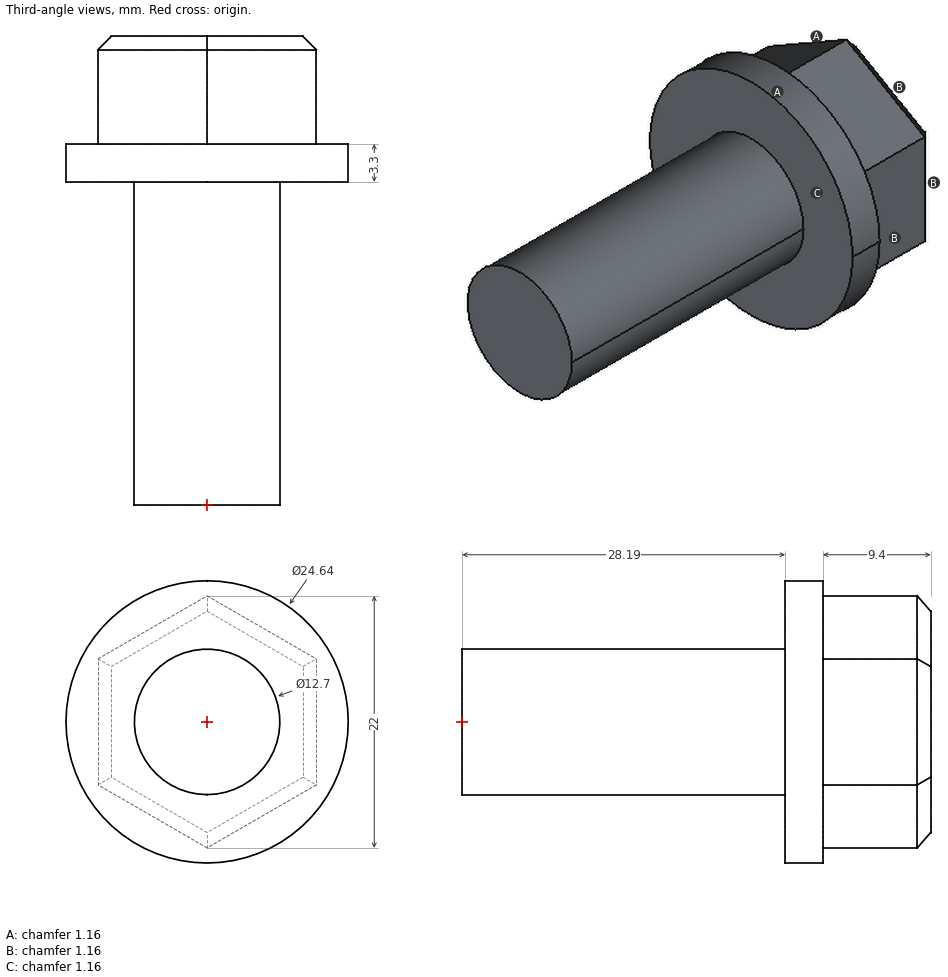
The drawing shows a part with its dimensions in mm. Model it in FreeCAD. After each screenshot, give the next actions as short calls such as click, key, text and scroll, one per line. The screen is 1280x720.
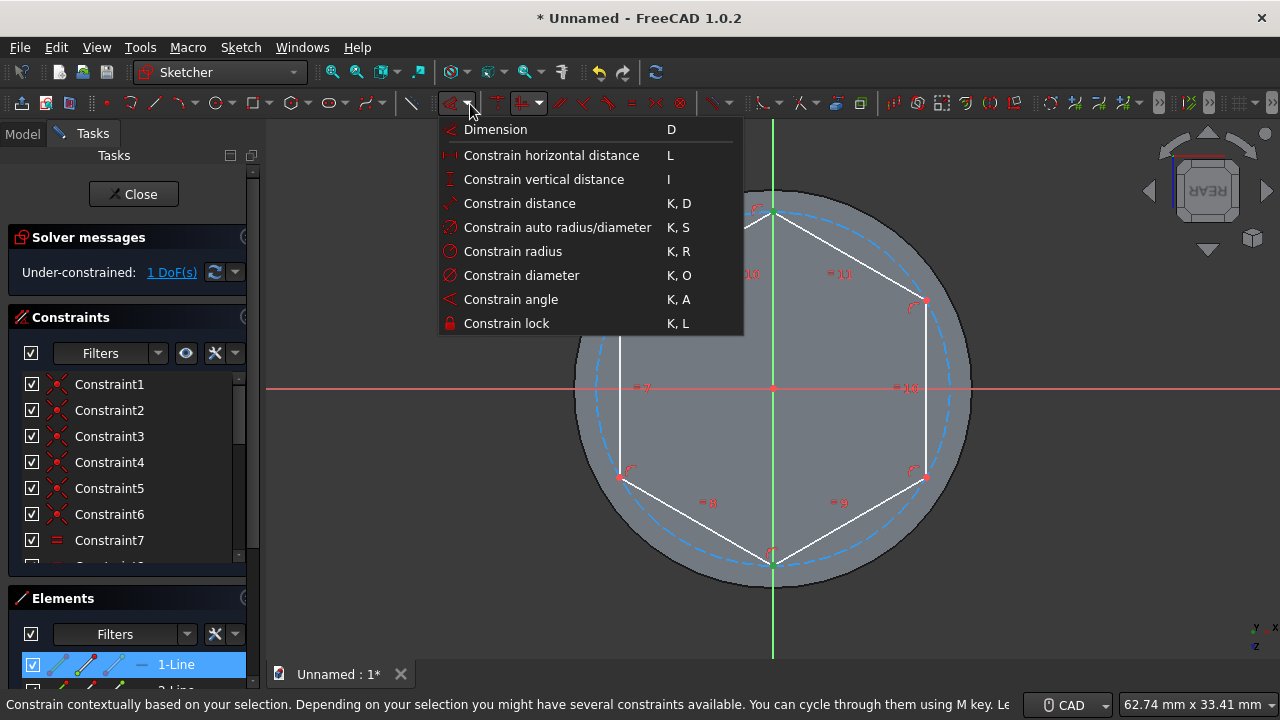
click(591, 179)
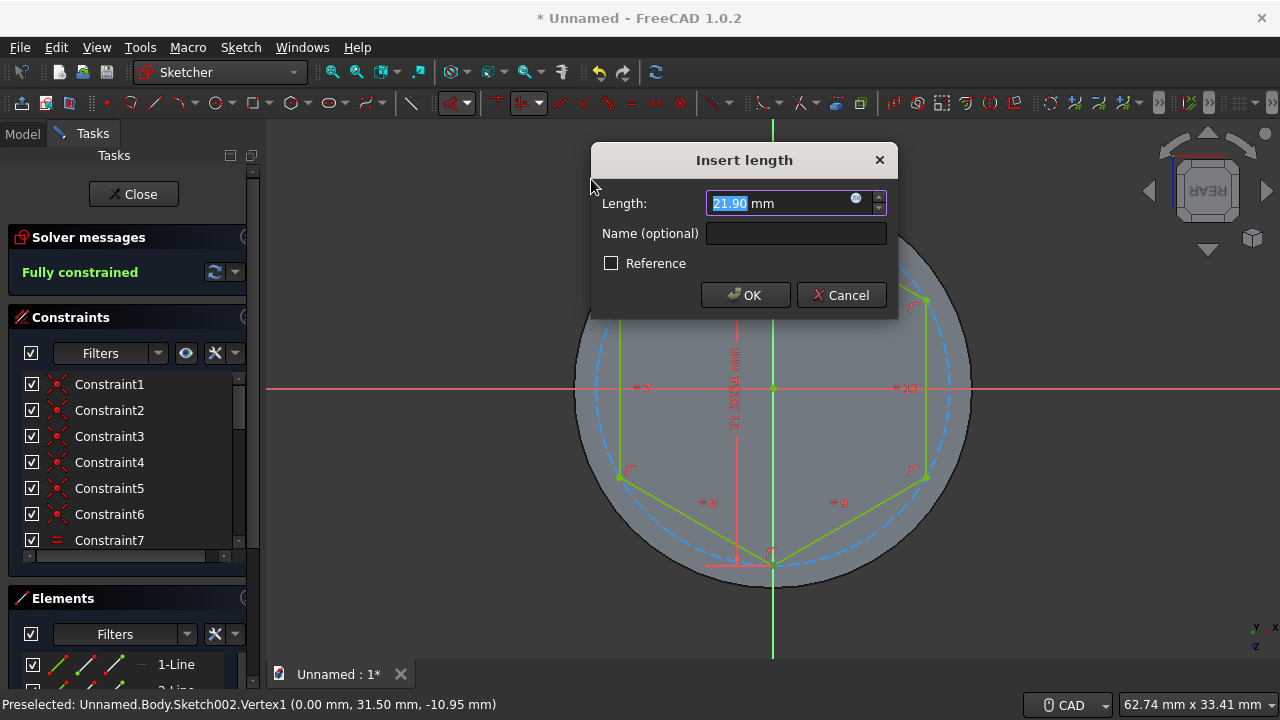
text(22)
key(Return)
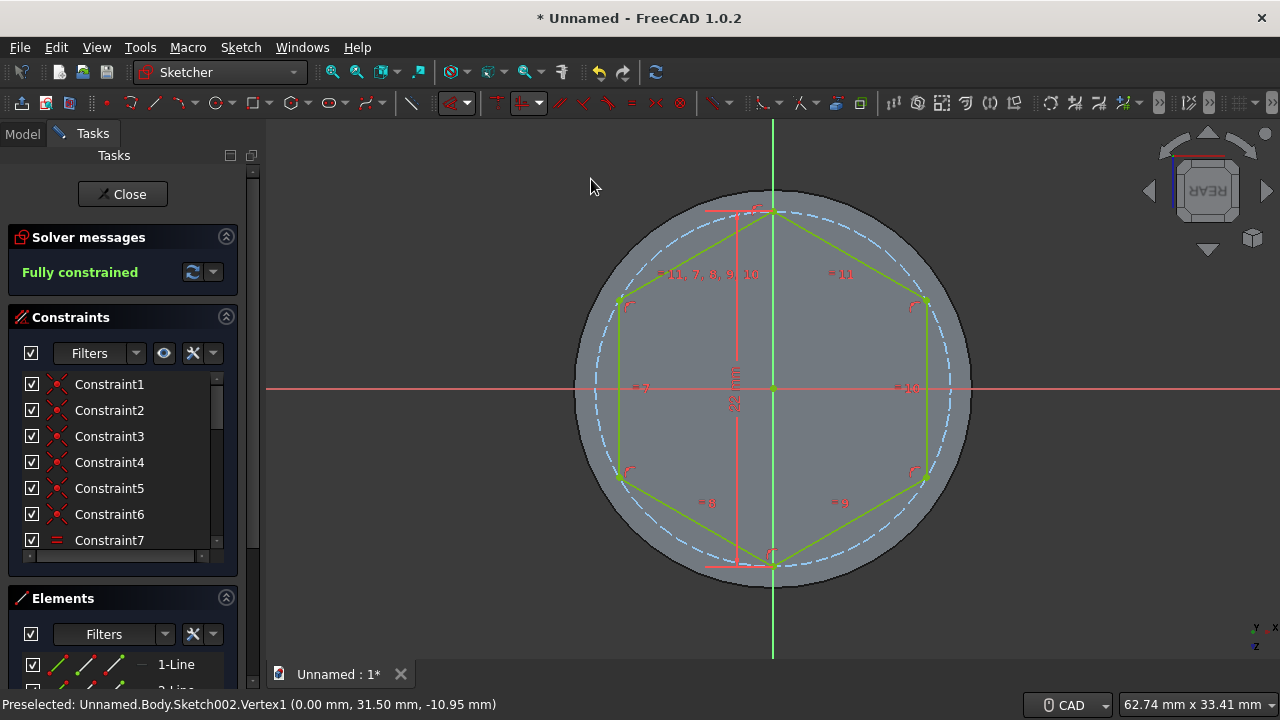
click(123, 194)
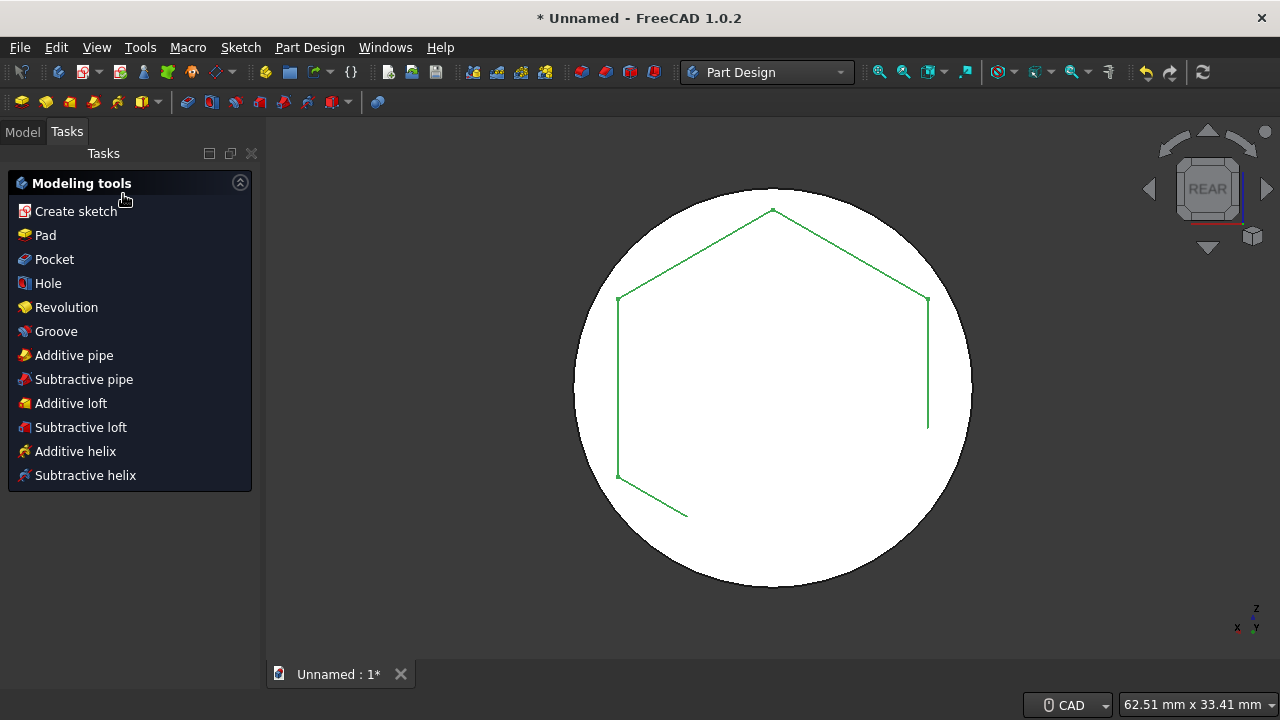
click(22, 102)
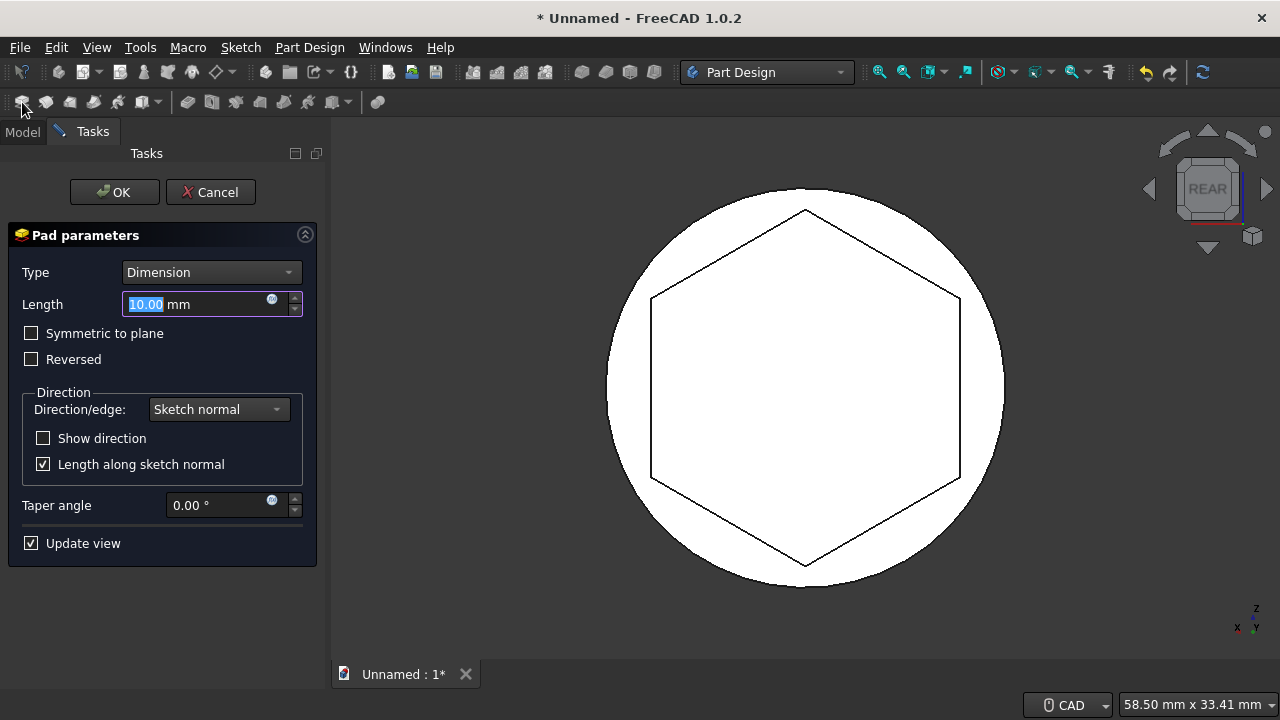
text(9.4)
key(Tab)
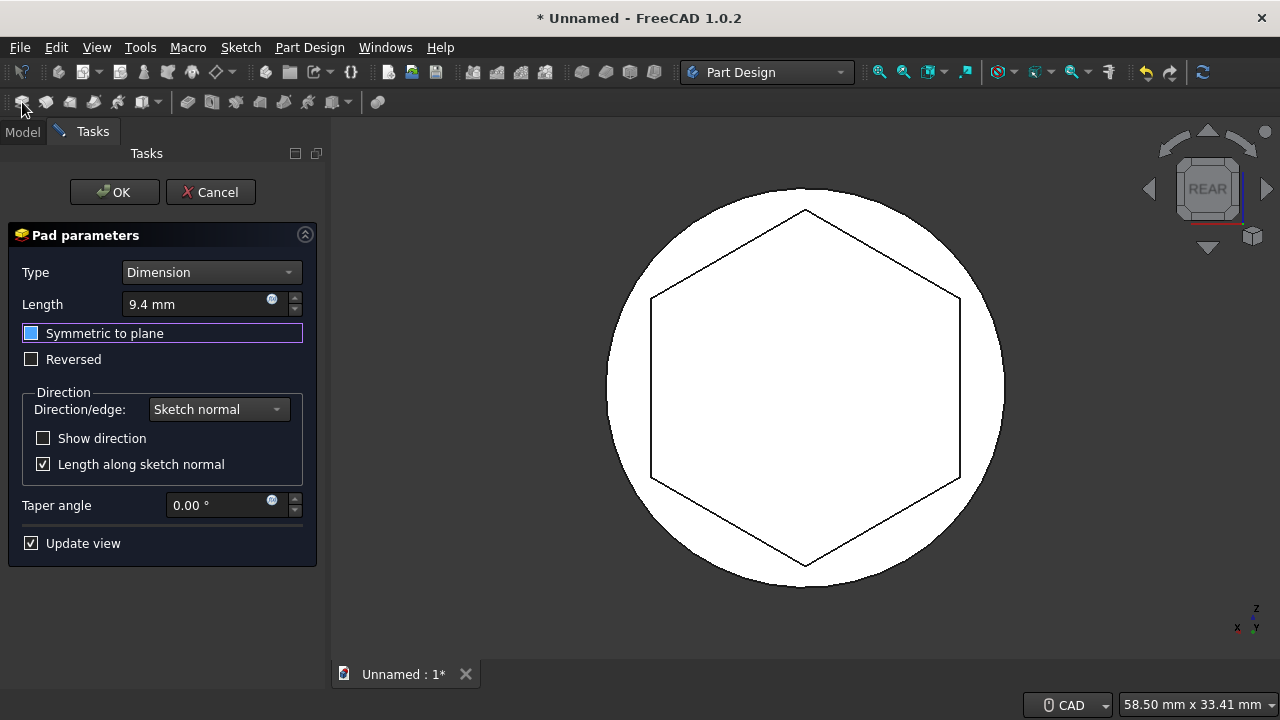
click(115, 192)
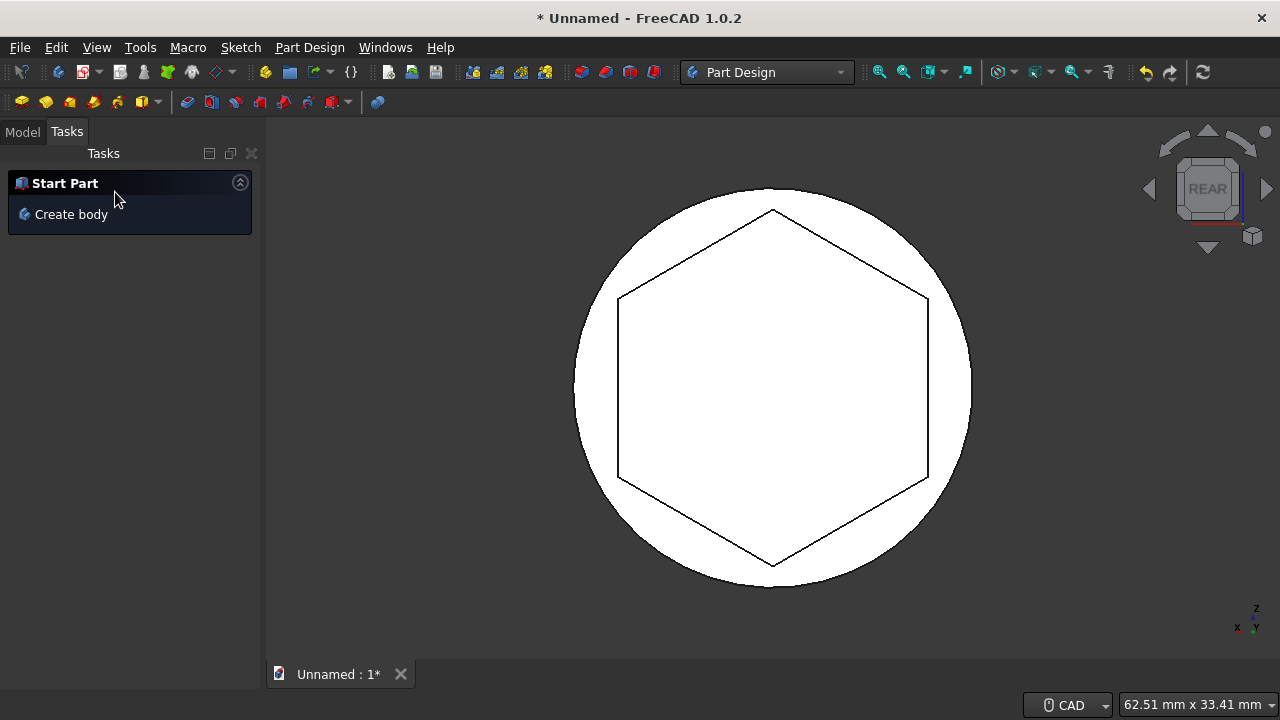
click(928, 387)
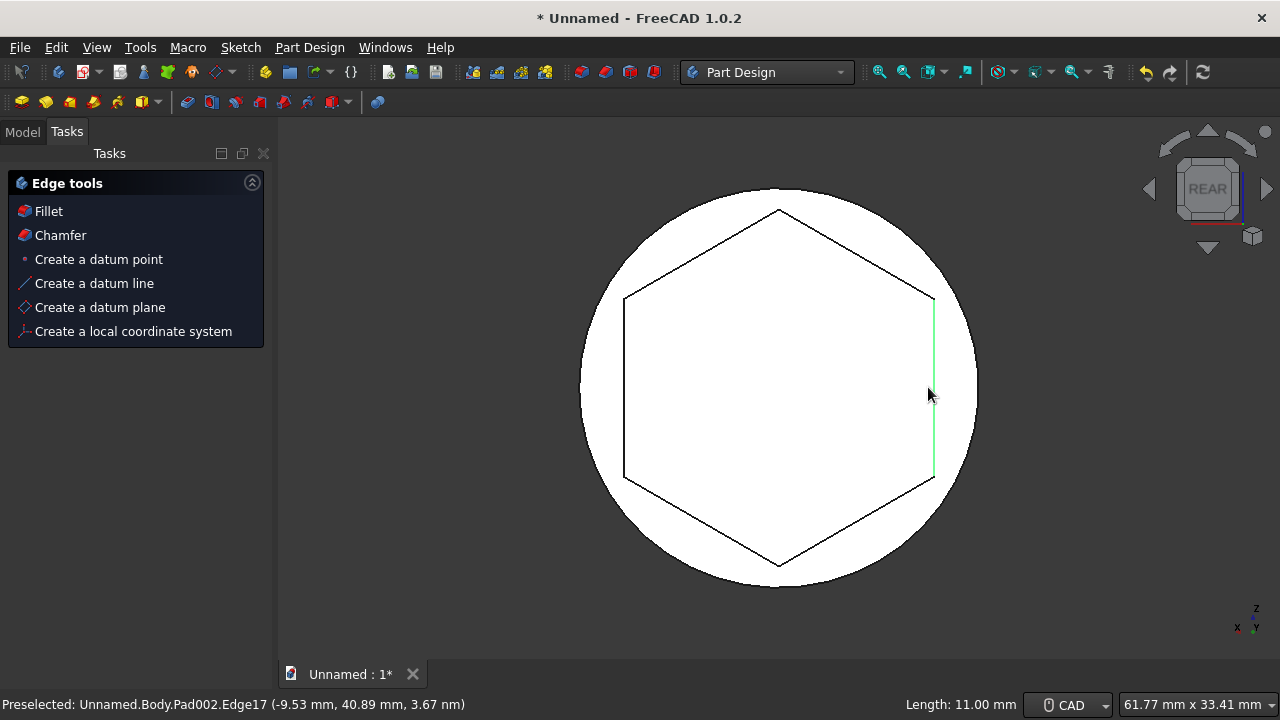
key(0)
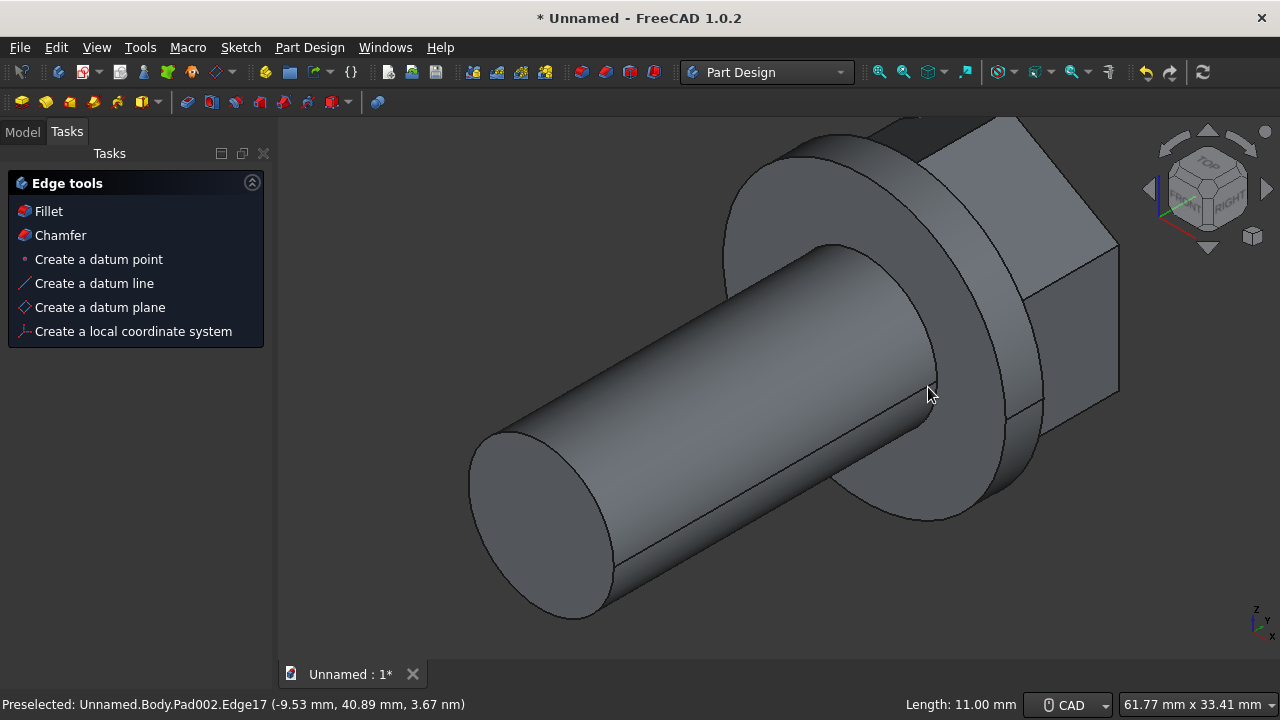
click(880, 72)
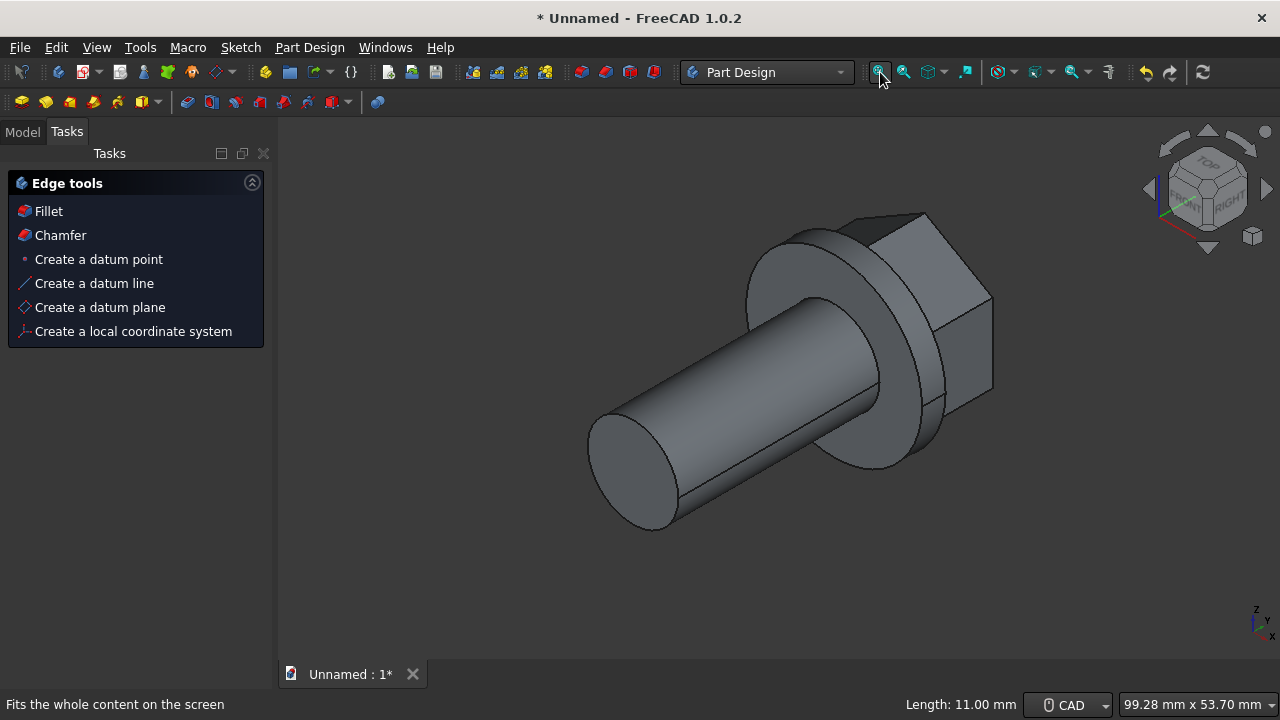
key(2)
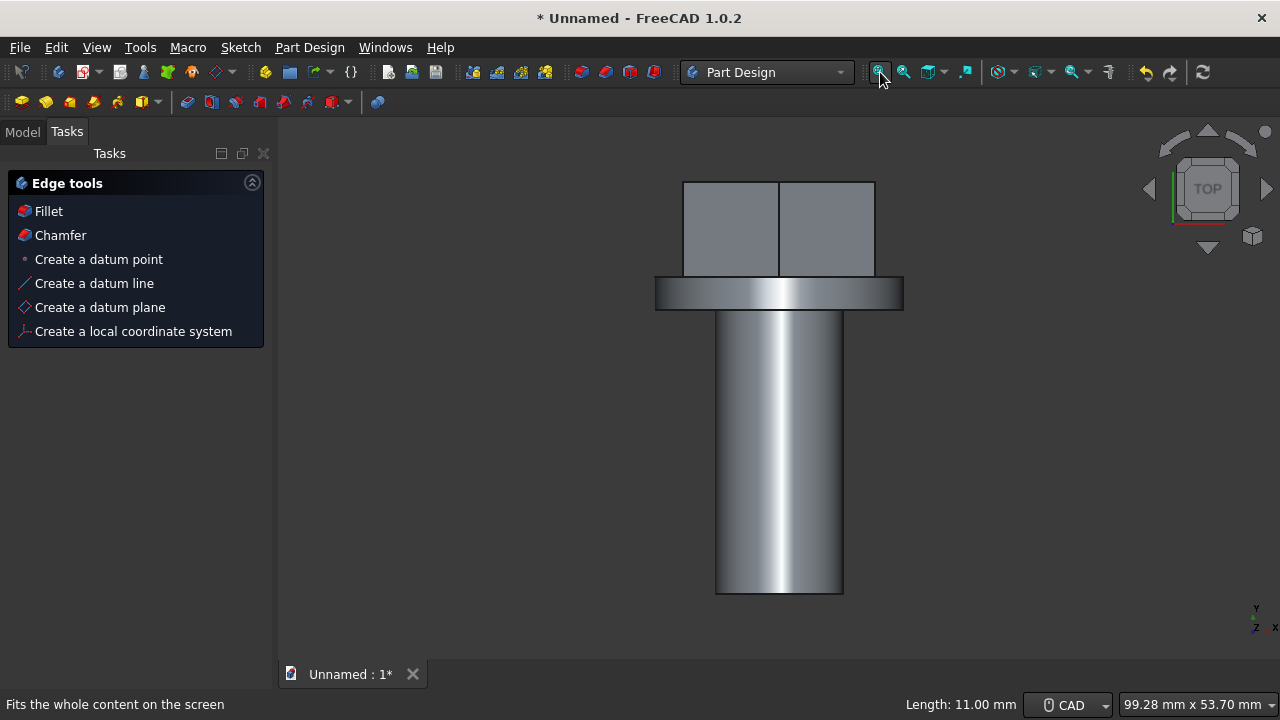
click(731, 181, ctrl)